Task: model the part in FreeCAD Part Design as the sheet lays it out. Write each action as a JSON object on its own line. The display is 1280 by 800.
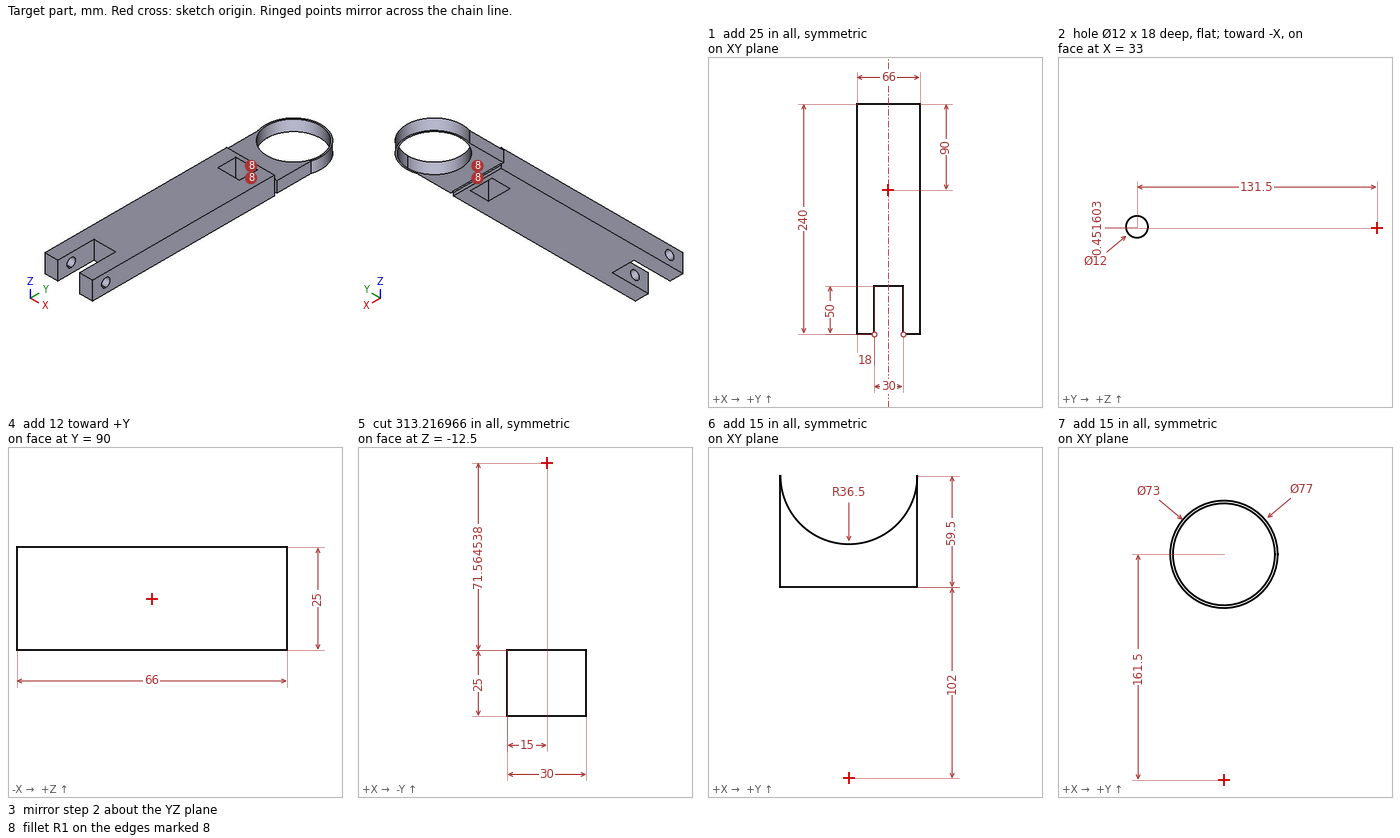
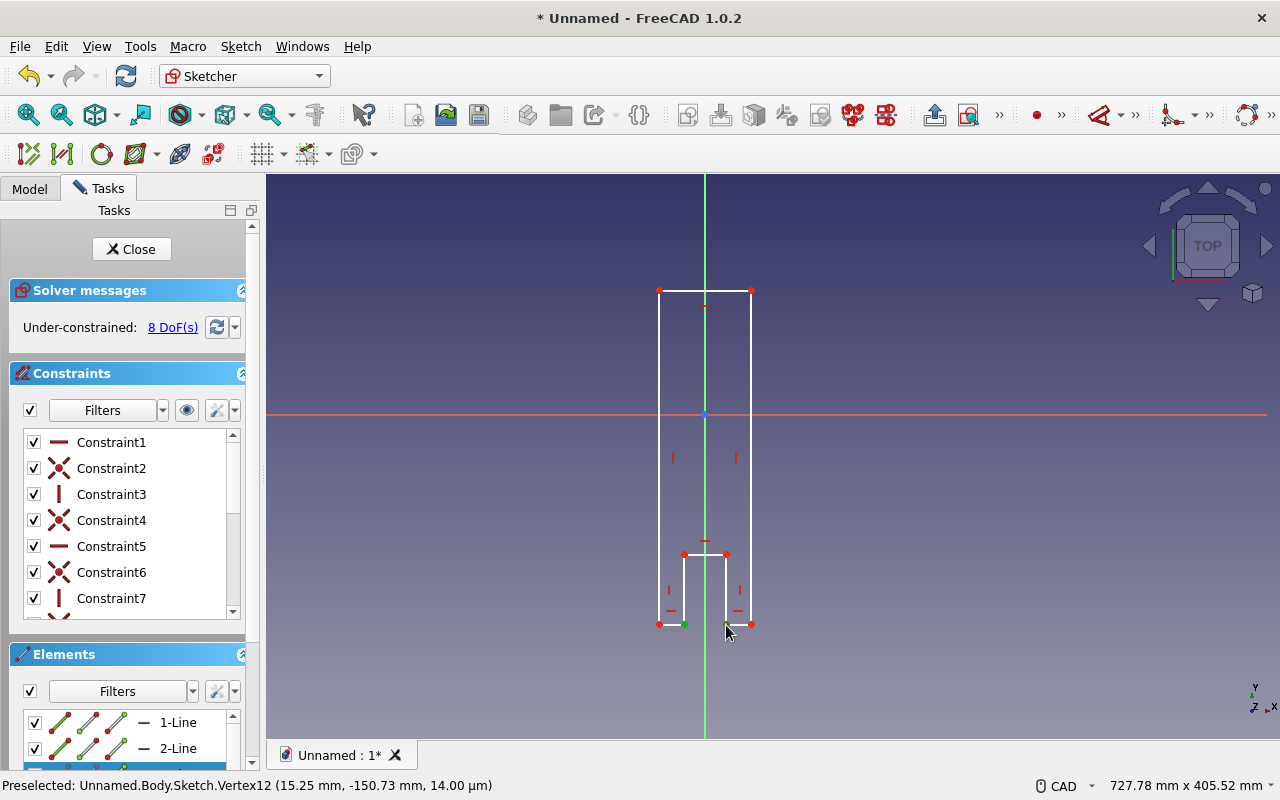
{"action": "left_click", "coordinate": [705, 675]}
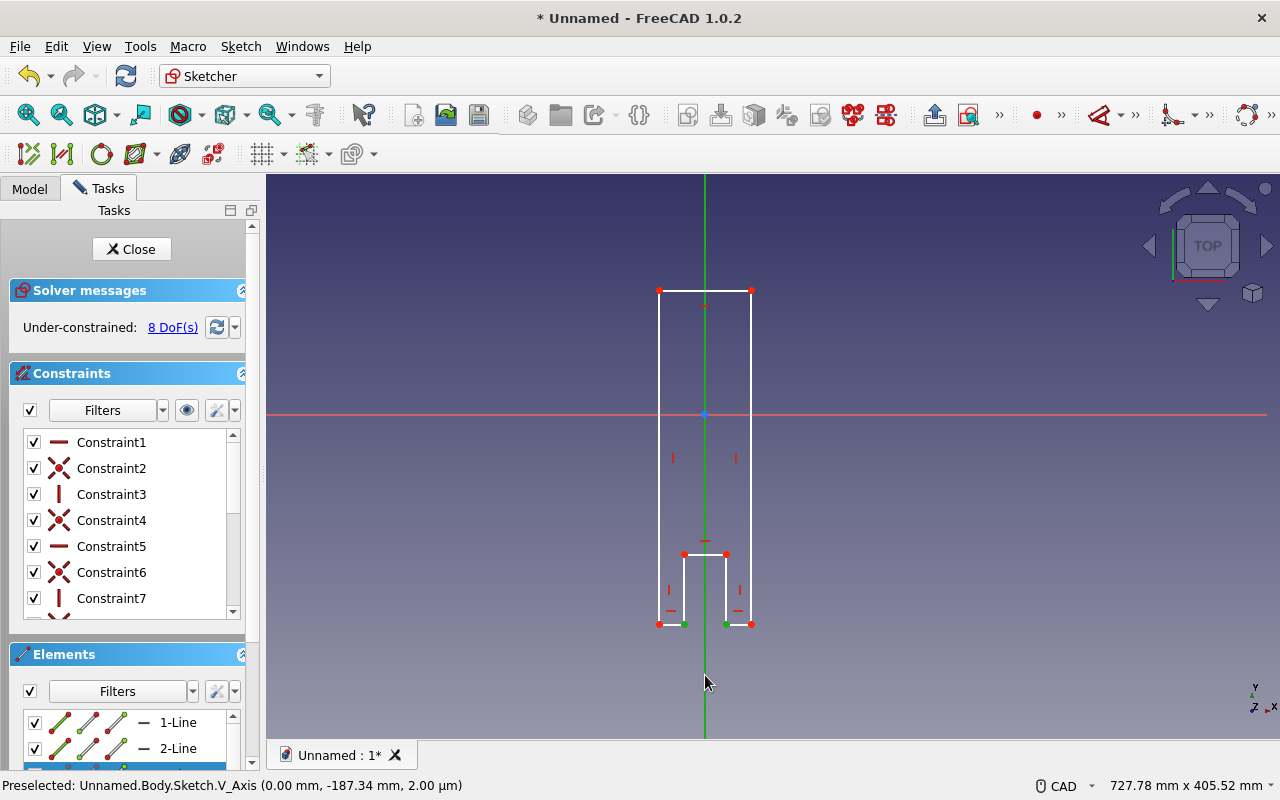
{"action": "key", "text": "s"}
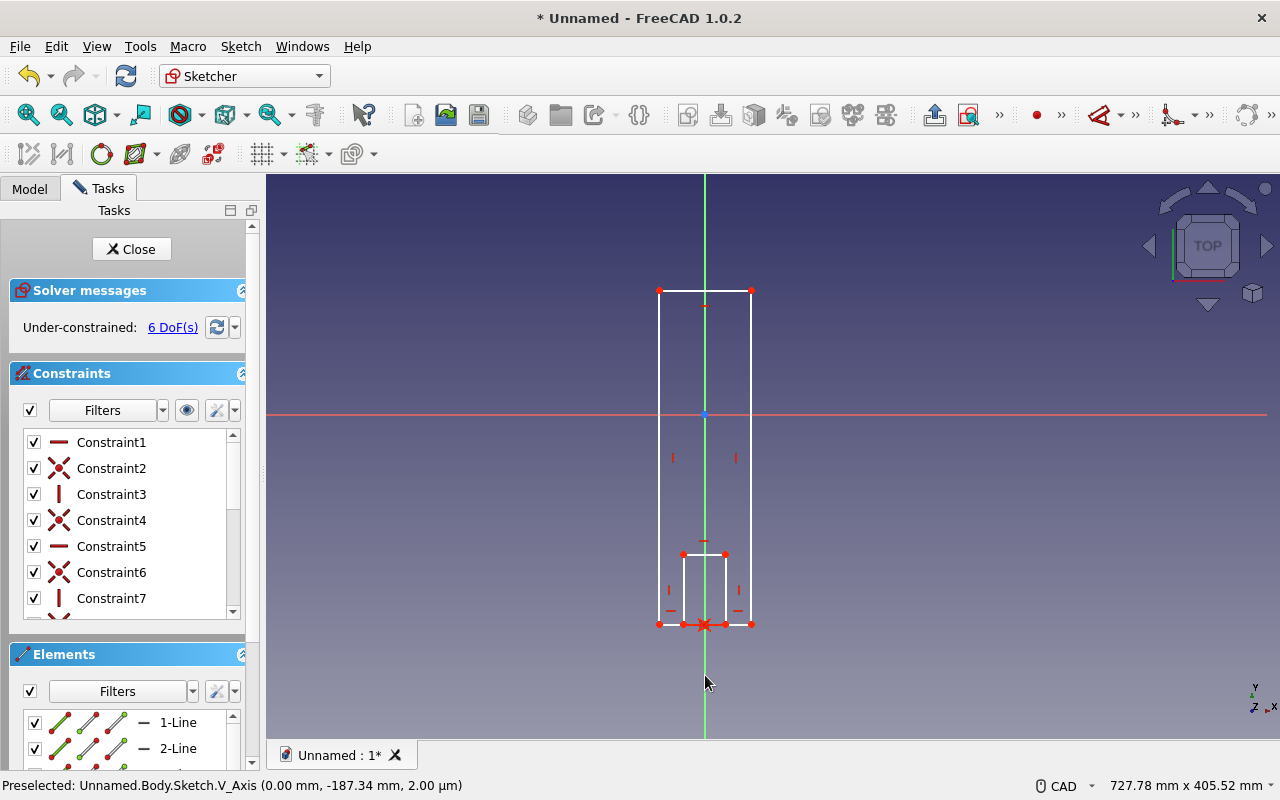
{"action": "key", "text": "d"}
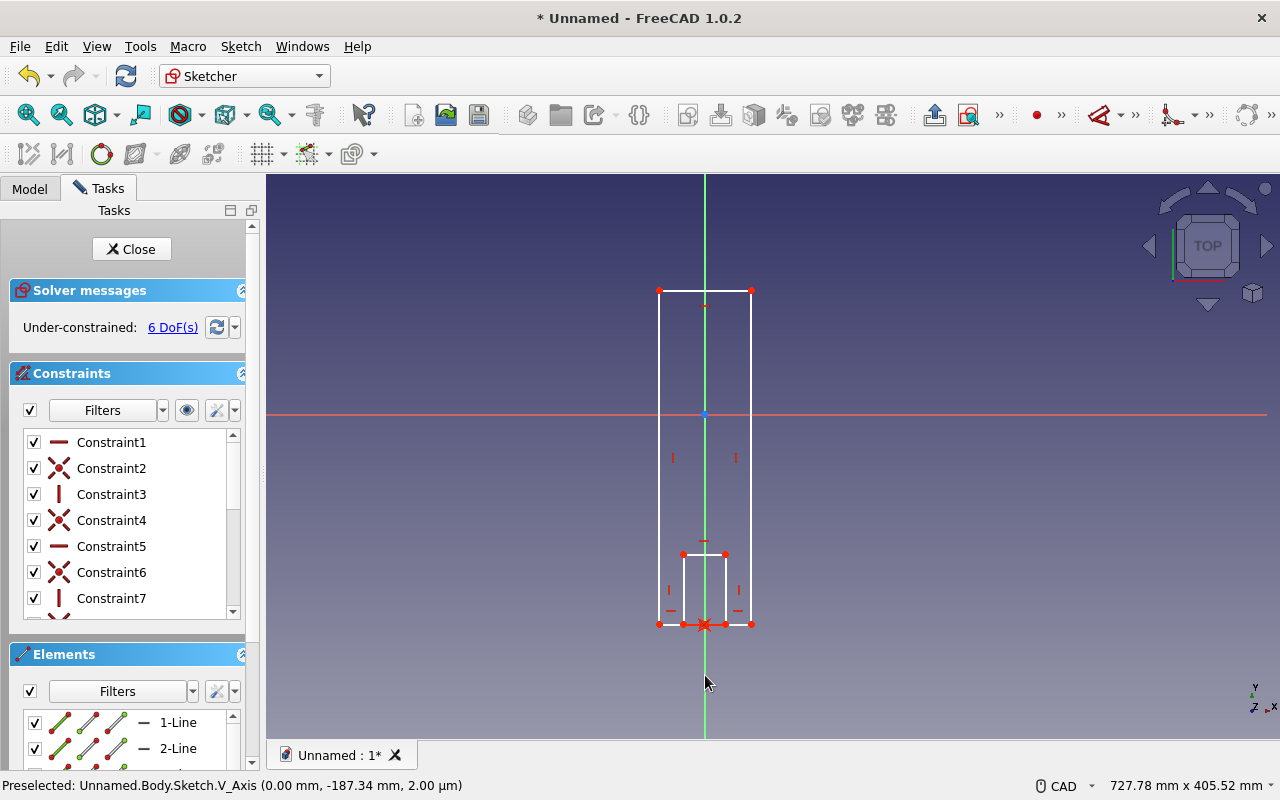
{"action": "left_click", "coordinate": [723, 291]}
{"action": "left_click", "coordinate": [684, 257]}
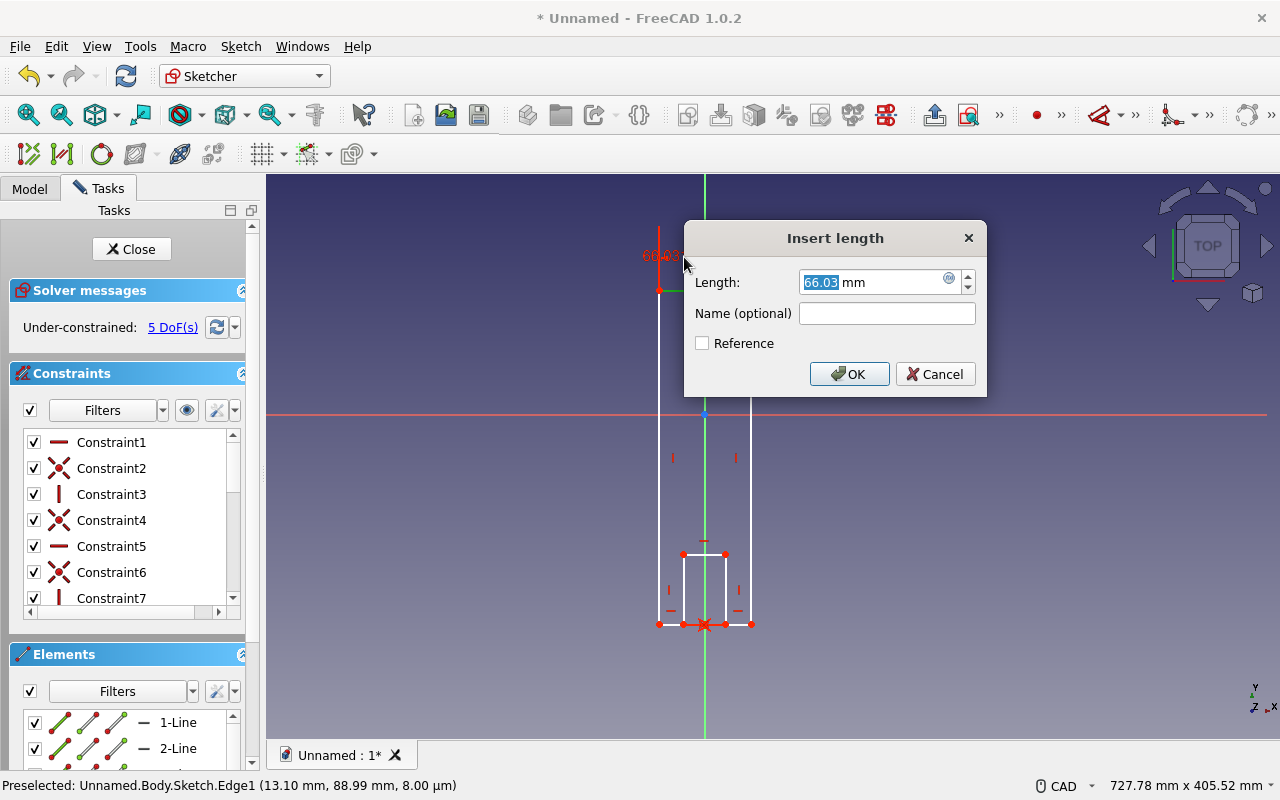
{"action": "type", "text": "66"}
{"action": "key", "text": "Return"}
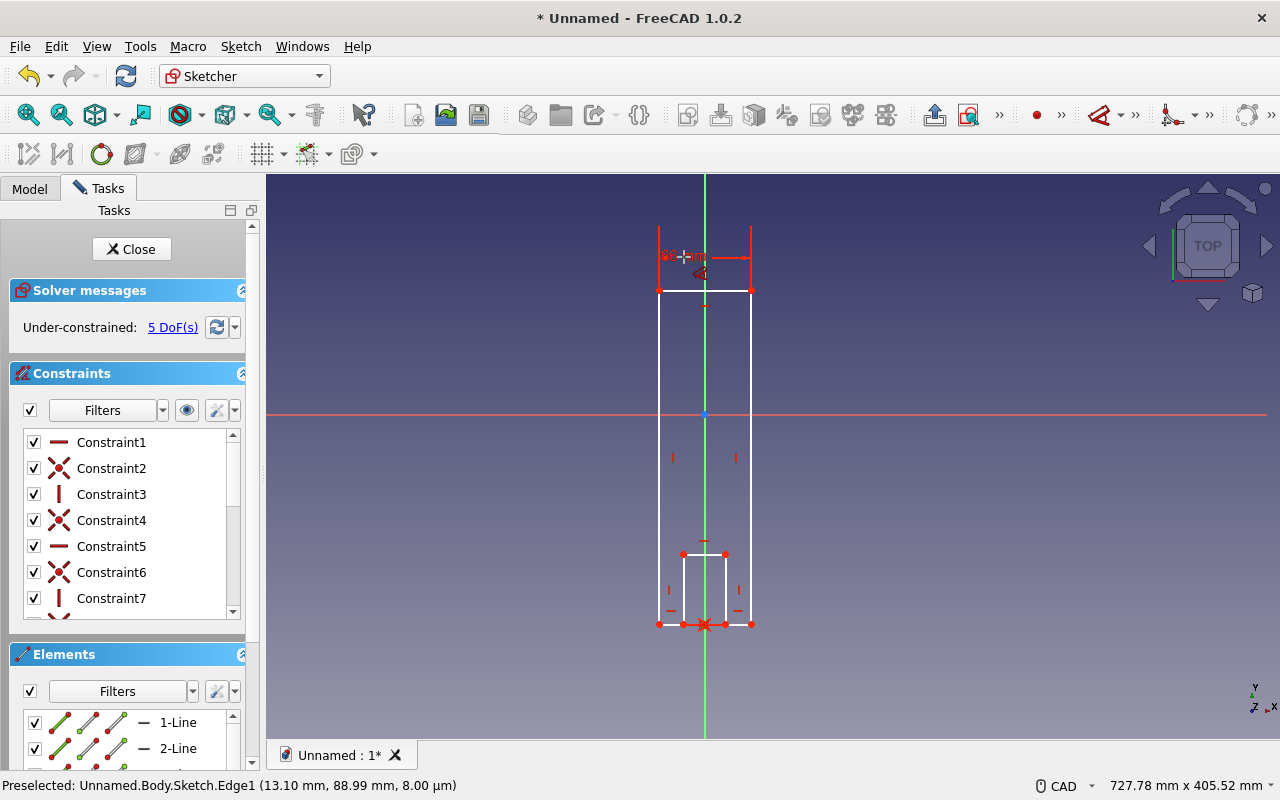
{"action": "scroll", "coordinate": [669, 625], "scroll_direction": "up", "scroll_amount": 3}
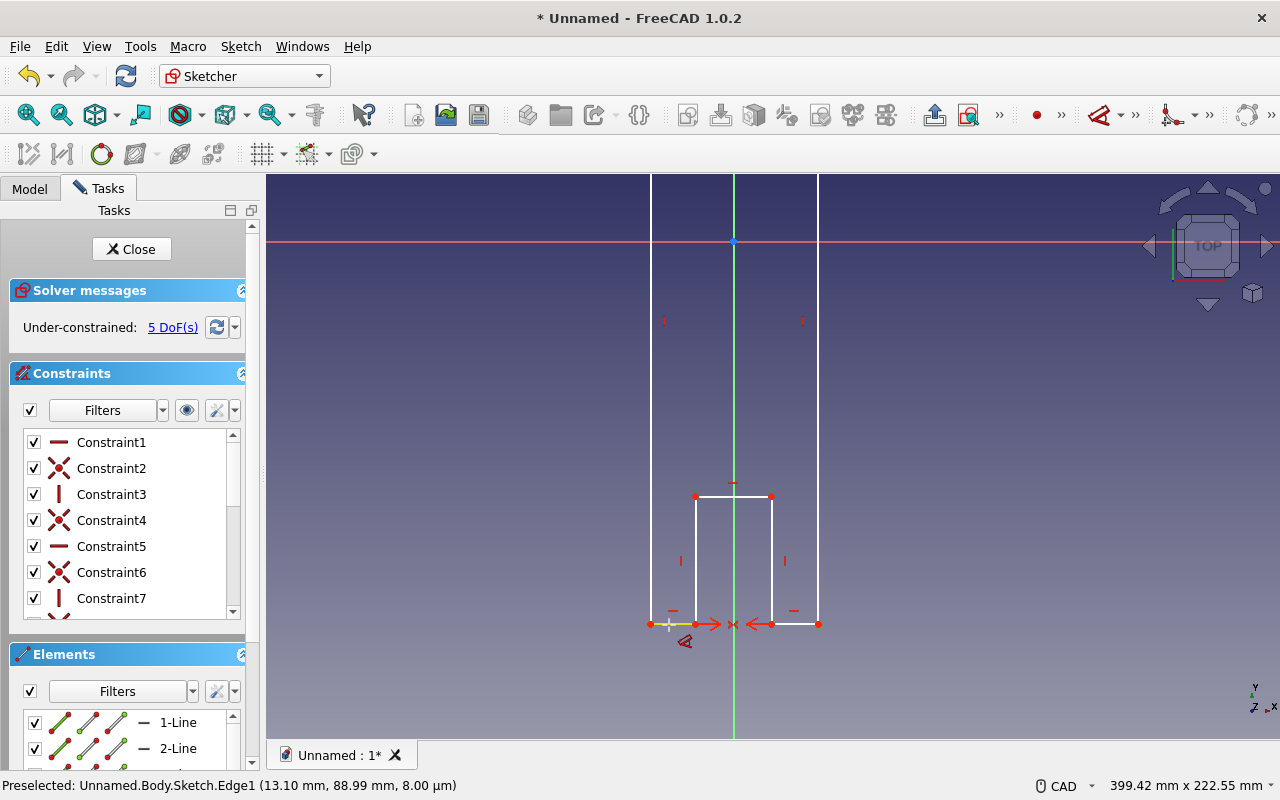
{"action": "left_click", "coordinate": [669, 624]}
{"action": "left_click", "coordinate": [673, 658]}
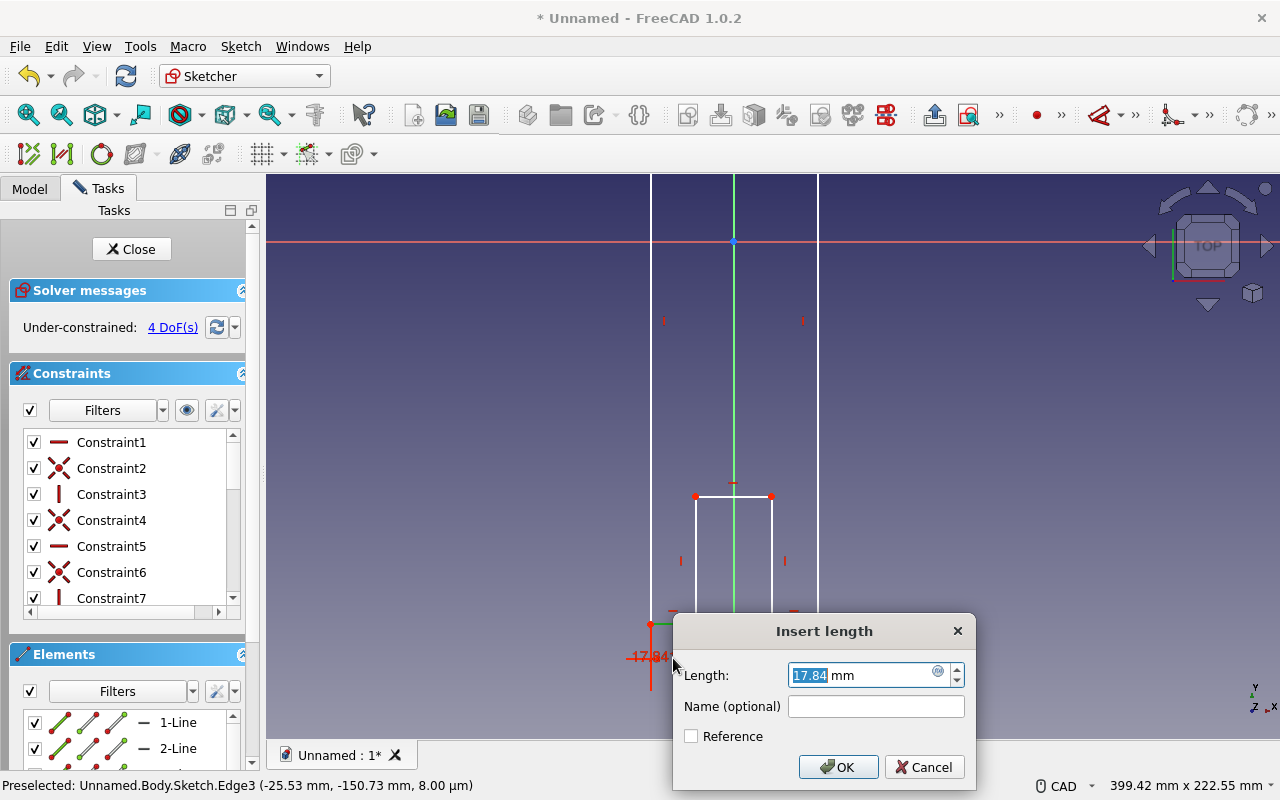
{"action": "type", "text": "18"}
{"action": "key", "text": "Return"}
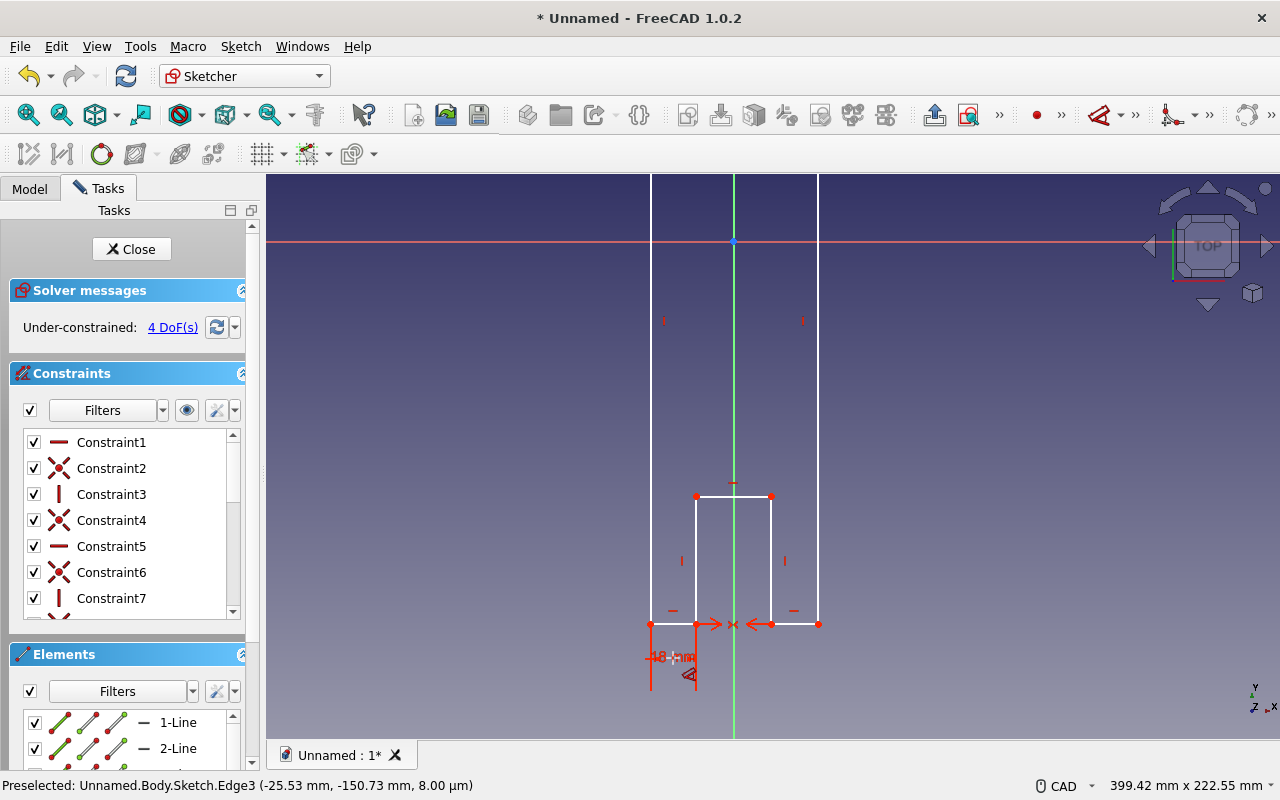
{"action": "left_click", "coordinate": [696, 586]}
{"action": "left_click", "coordinate": [754, 561]}